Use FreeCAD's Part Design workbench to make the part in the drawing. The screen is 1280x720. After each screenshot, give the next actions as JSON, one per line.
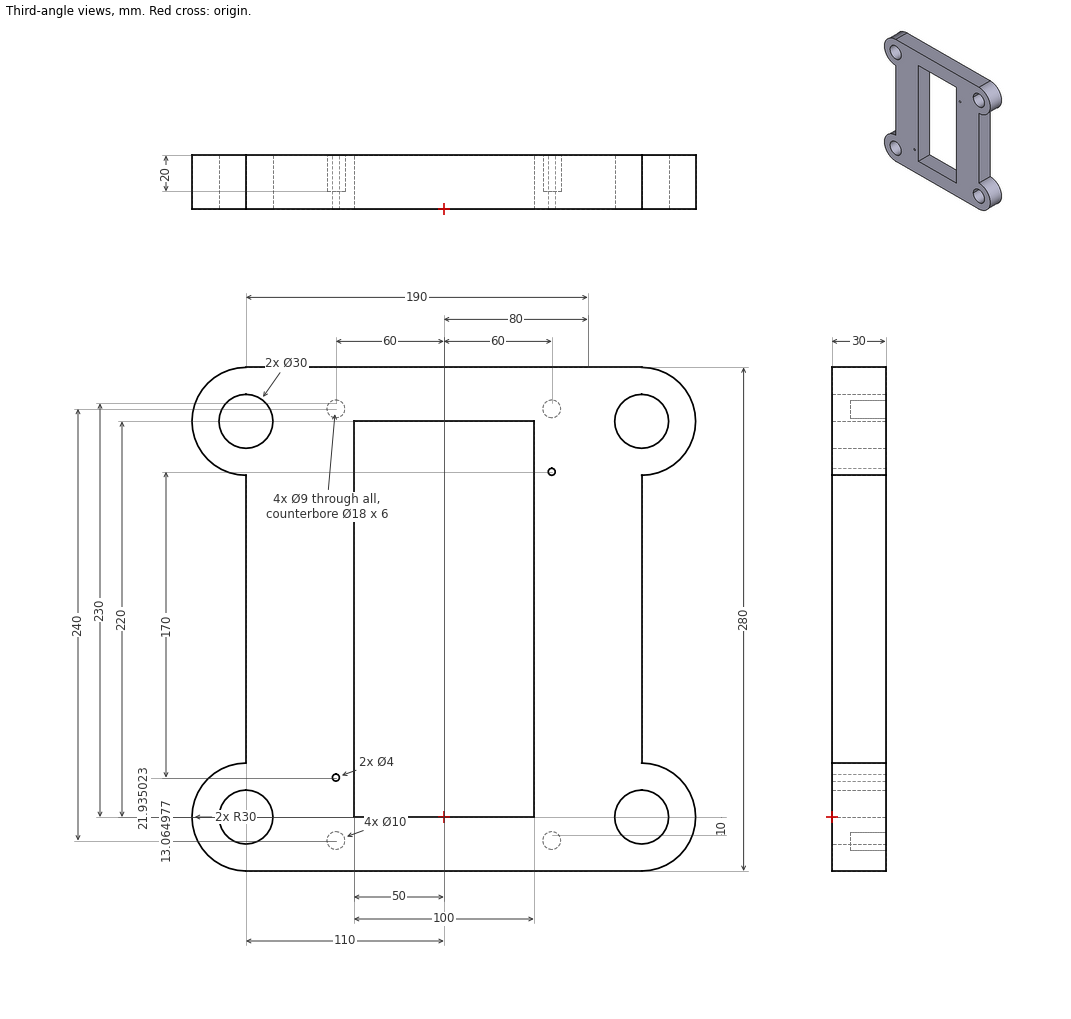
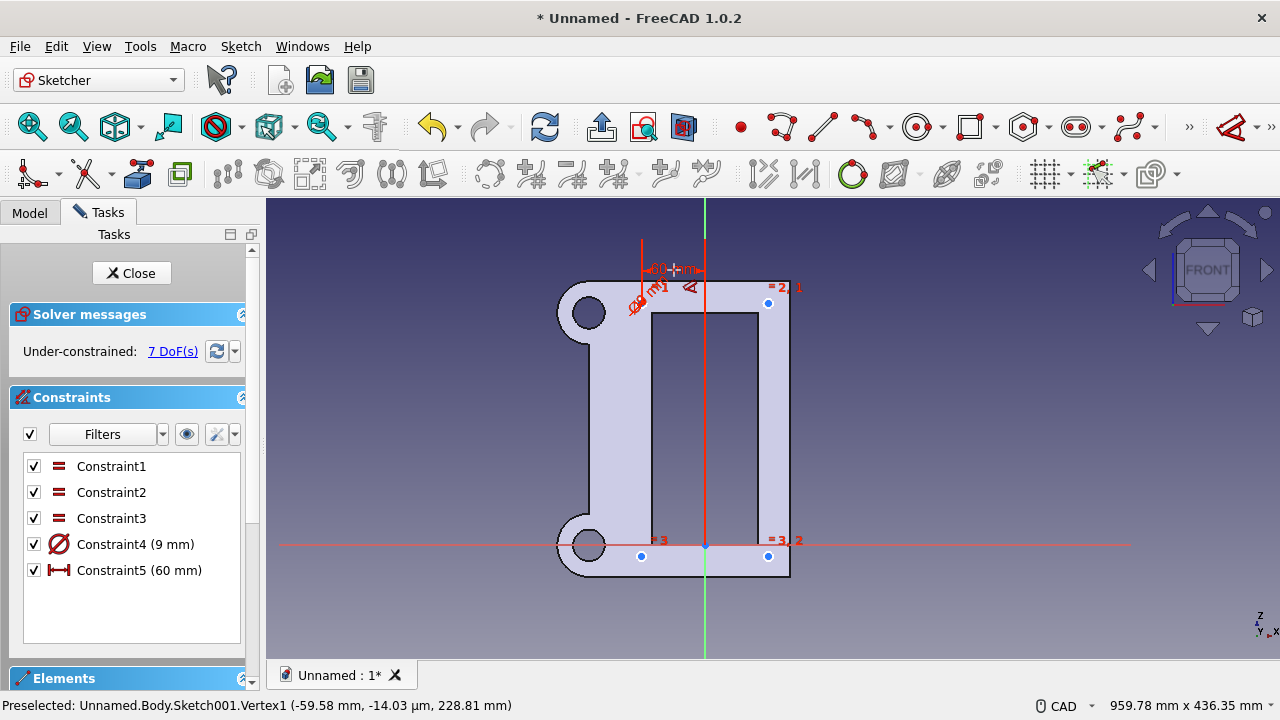
{"action": "left_click", "coordinate": [768, 304]}
{"action": "left_click", "coordinate": [751, 270]}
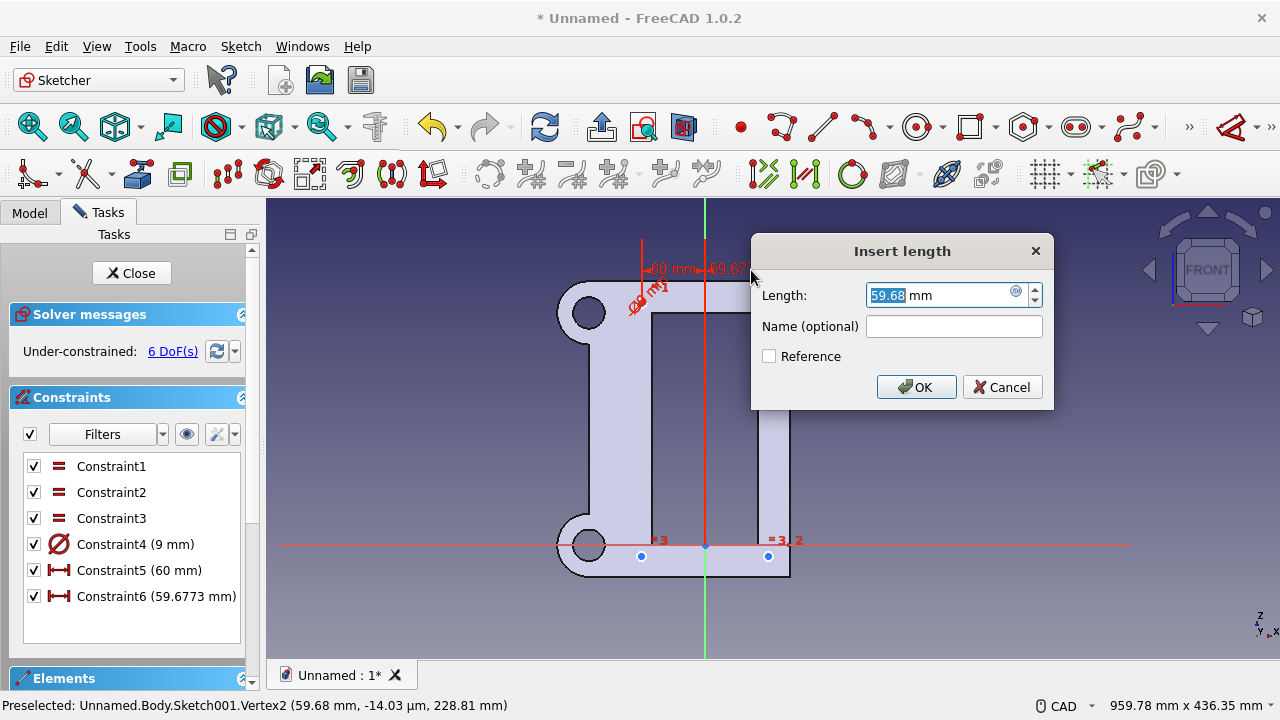
{"action": "type", "text": "60"}
{"action": "key", "text": "Return"}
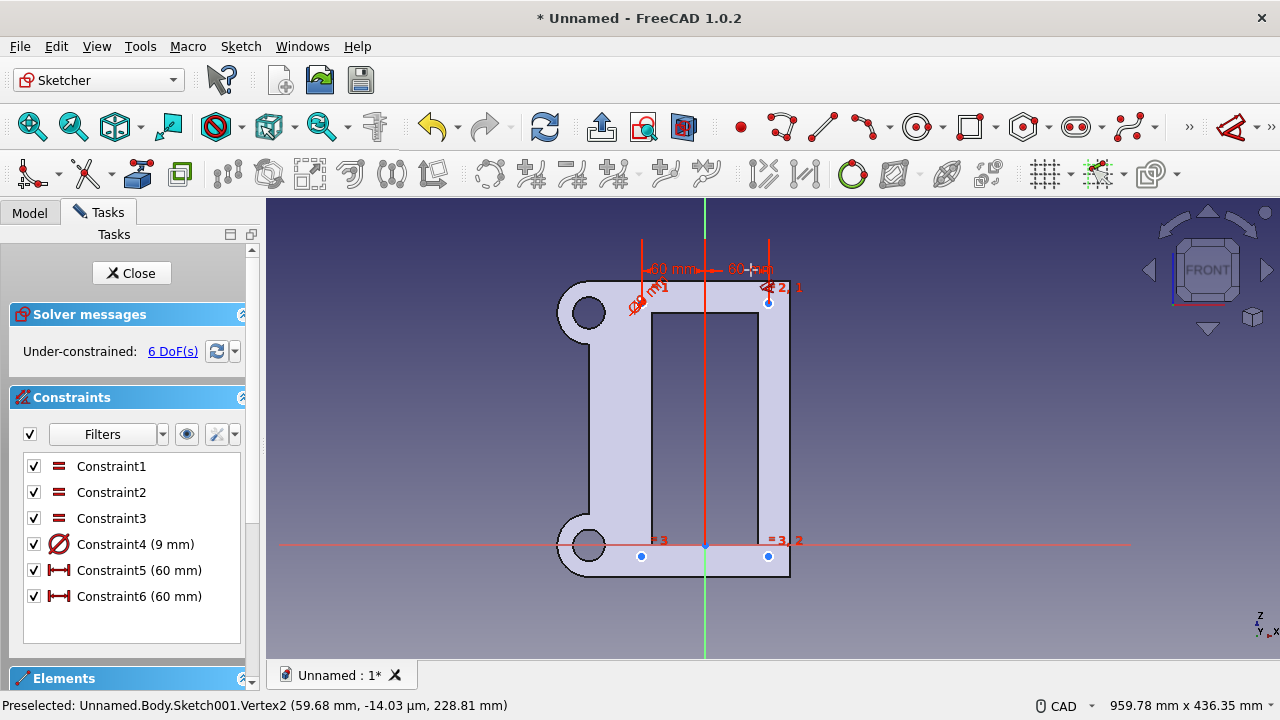
{"action": "left_click", "coordinate": [768, 557]}
{"action": "left_click", "coordinate": [737, 591]}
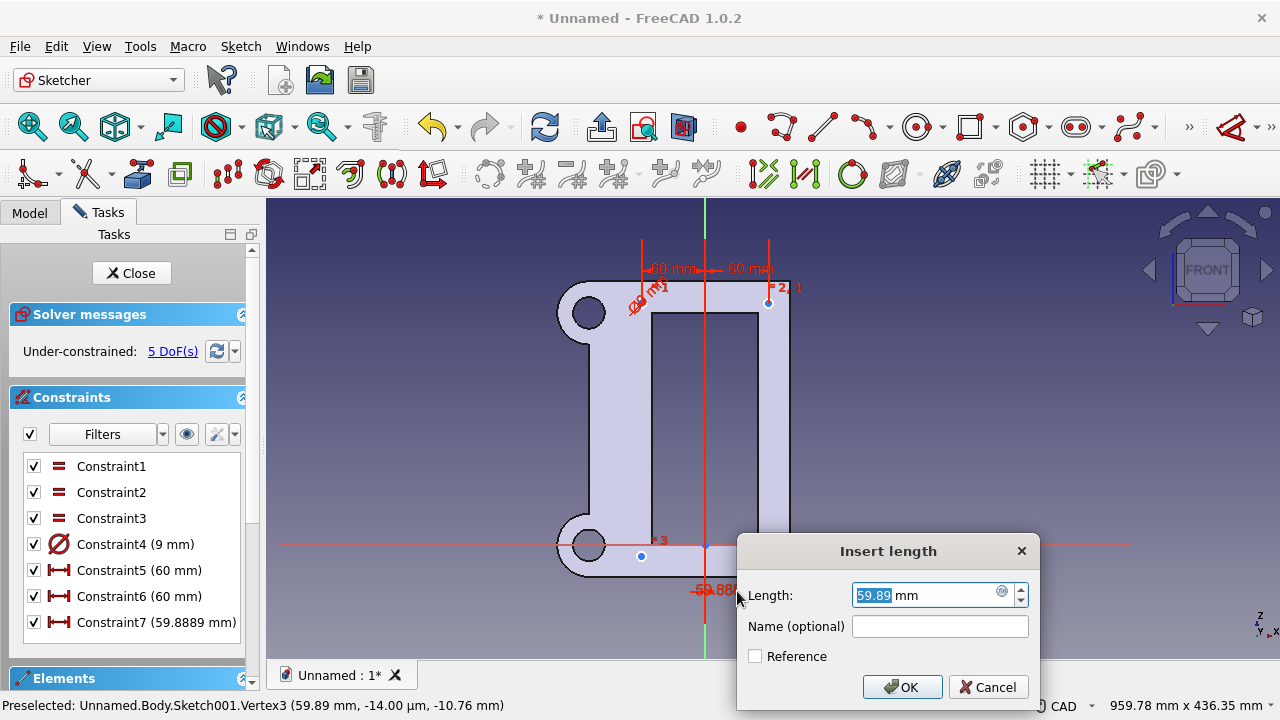
{"action": "type", "text": "60"}
{"action": "key", "text": "Return"}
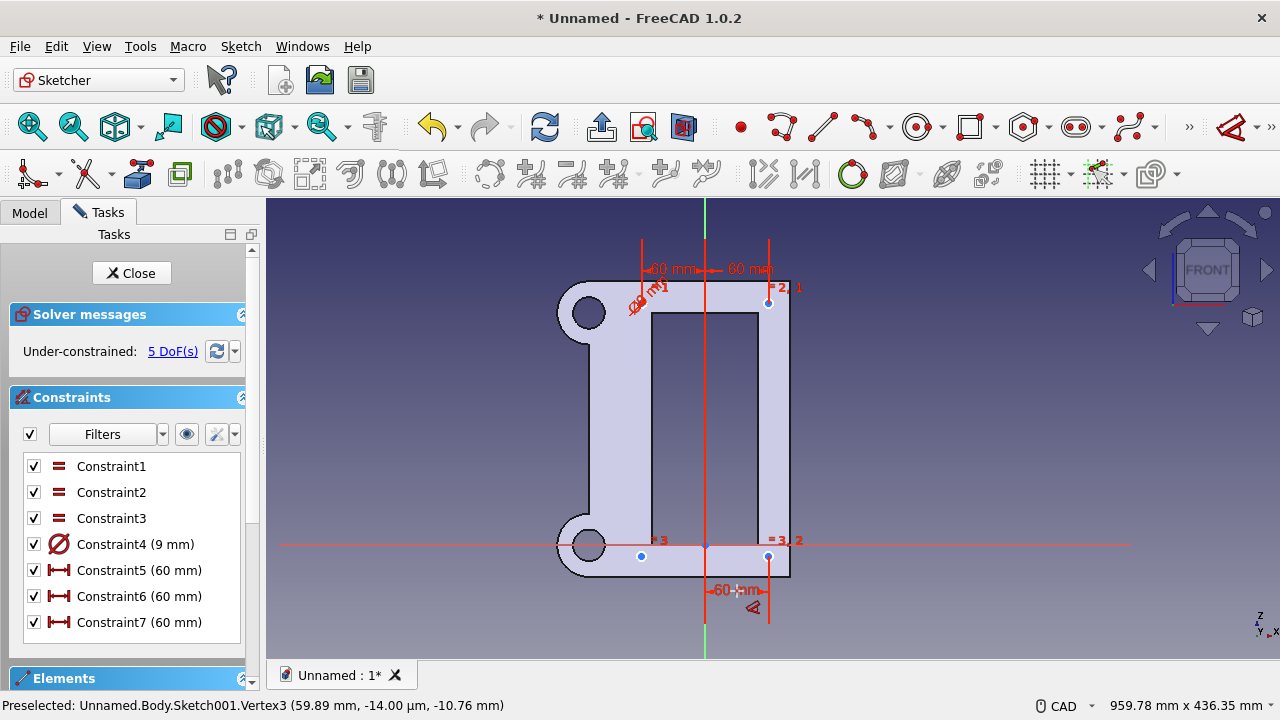
{"action": "scroll", "coordinate": [769, 557], "scroll_direction": "up", "scroll_amount": 7}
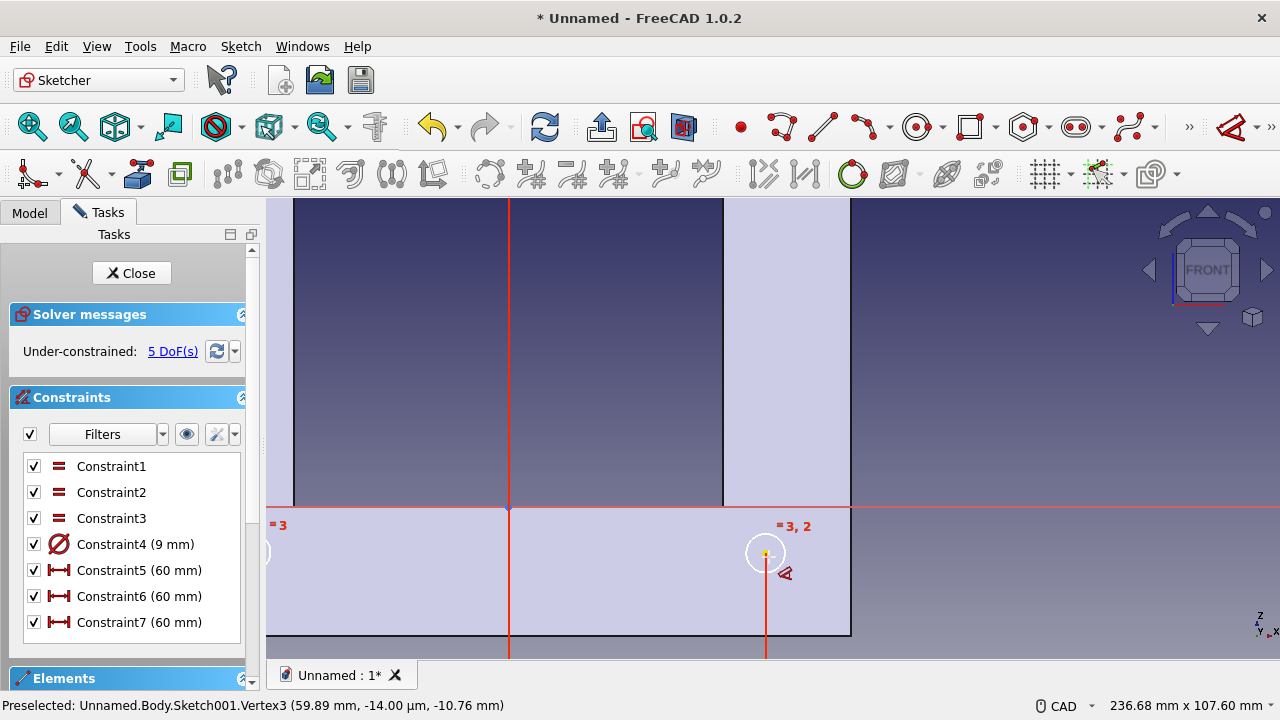
{"action": "left_click", "coordinate": [766, 553]}
{"action": "left_click", "coordinate": [800, 530]}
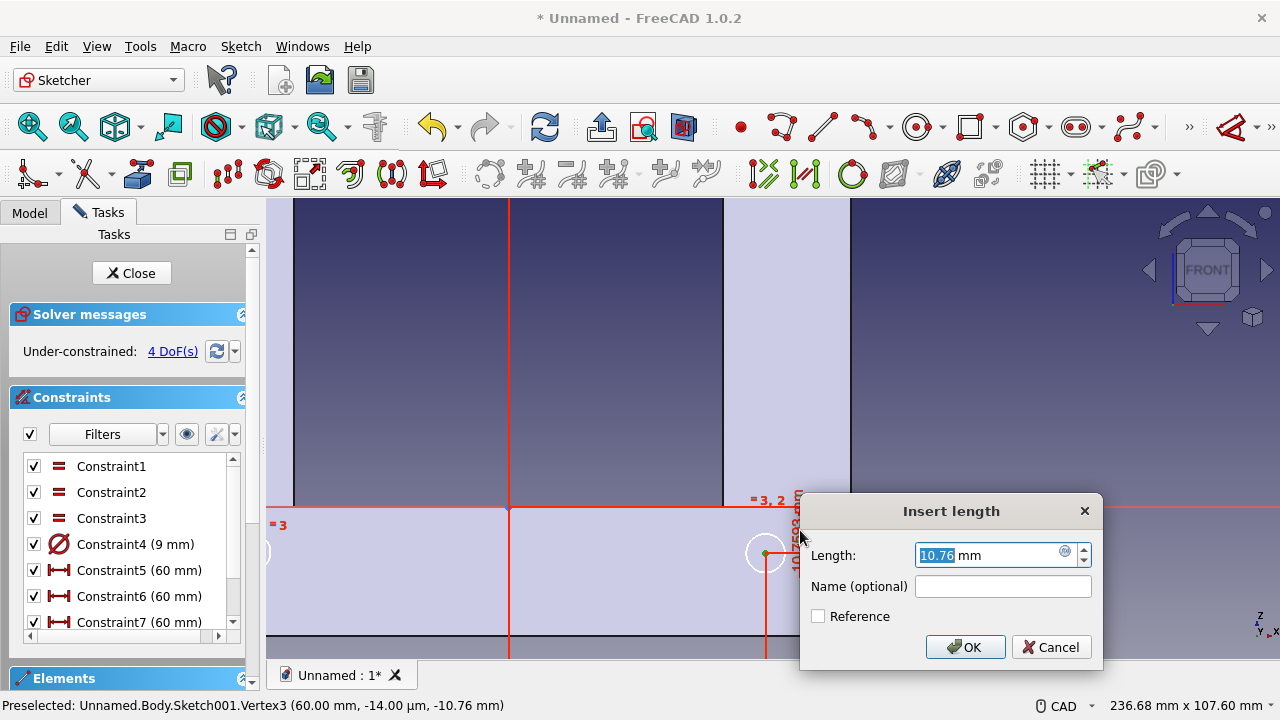
{"action": "type", "text": "10"}
{"action": "key", "text": "Return"}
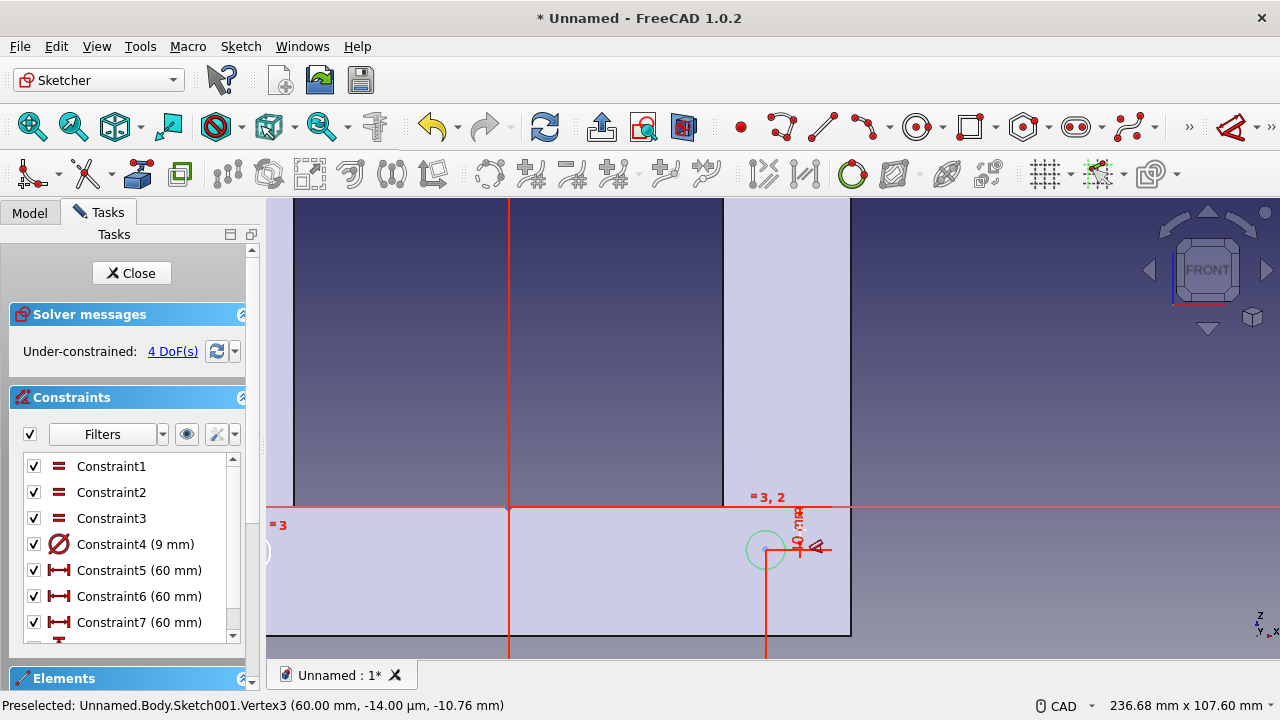
{"action": "scroll", "coordinate": [769, 557], "scroll_direction": "down", "scroll_amount": 7}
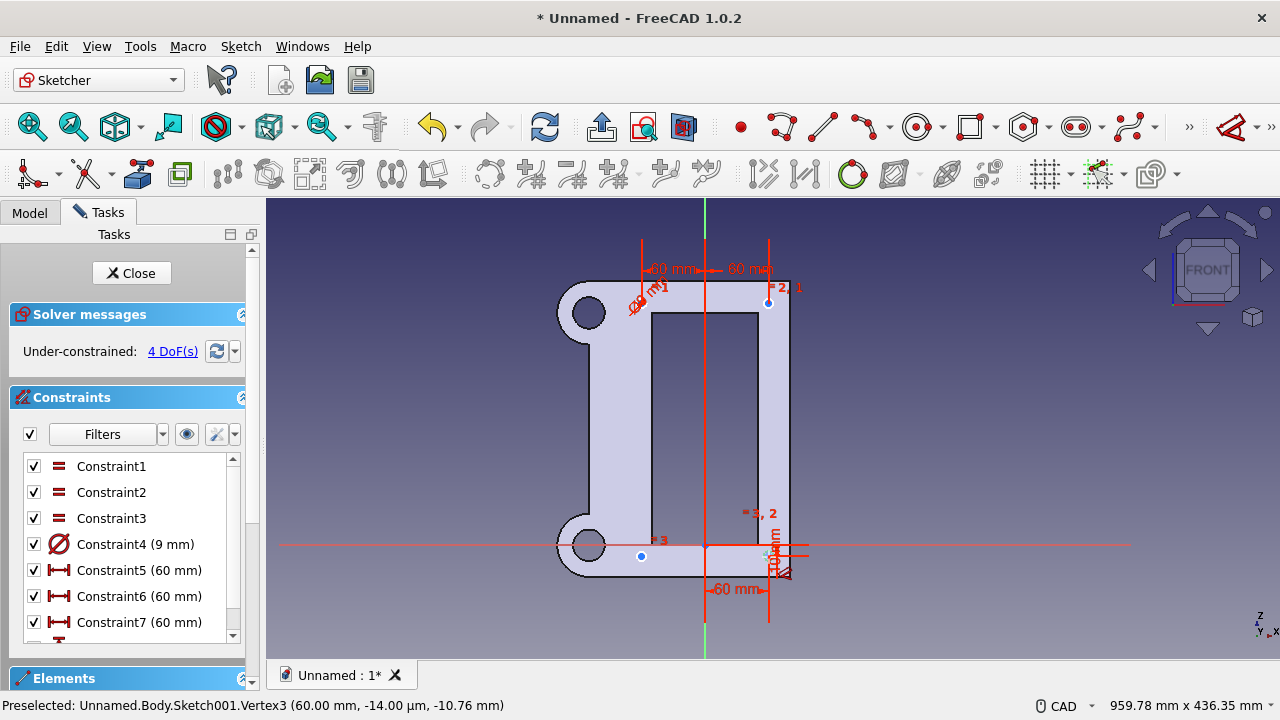
{"action": "left_click", "coordinate": [642, 556]}
{"action": "left_click", "coordinate": [659, 590]}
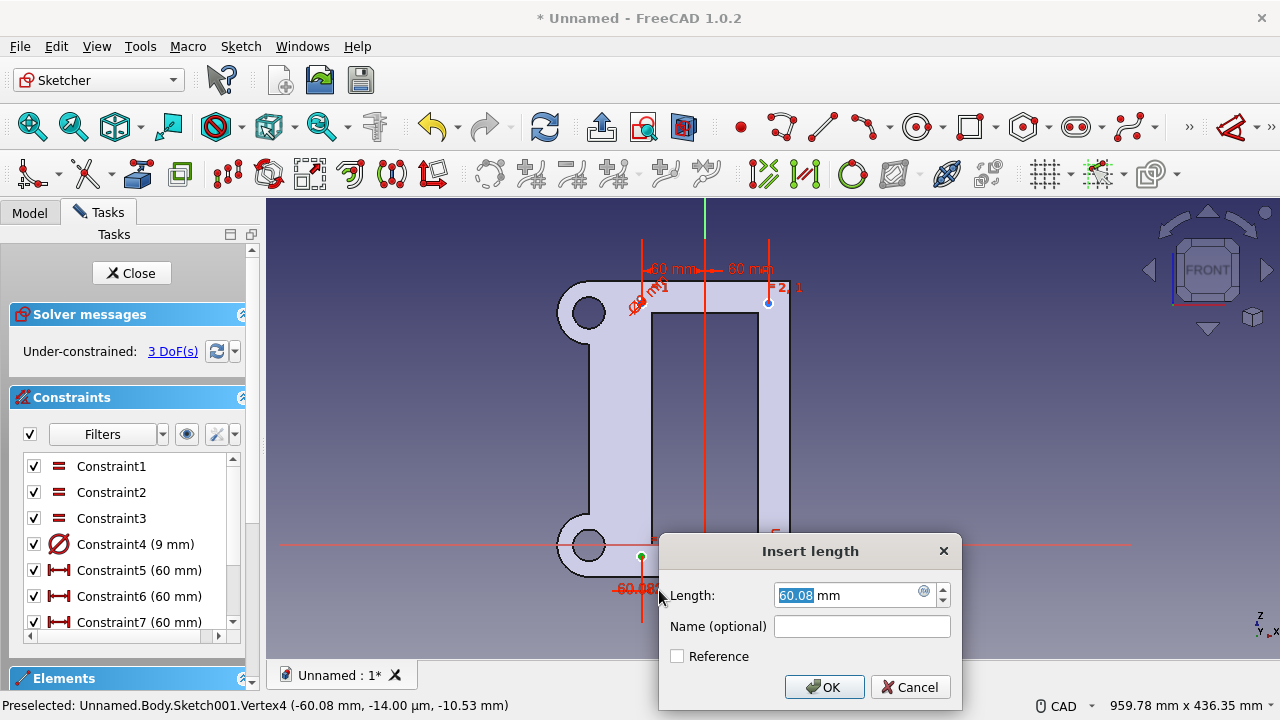
{"action": "type", "text": "60"}
{"action": "key", "text": "Return"}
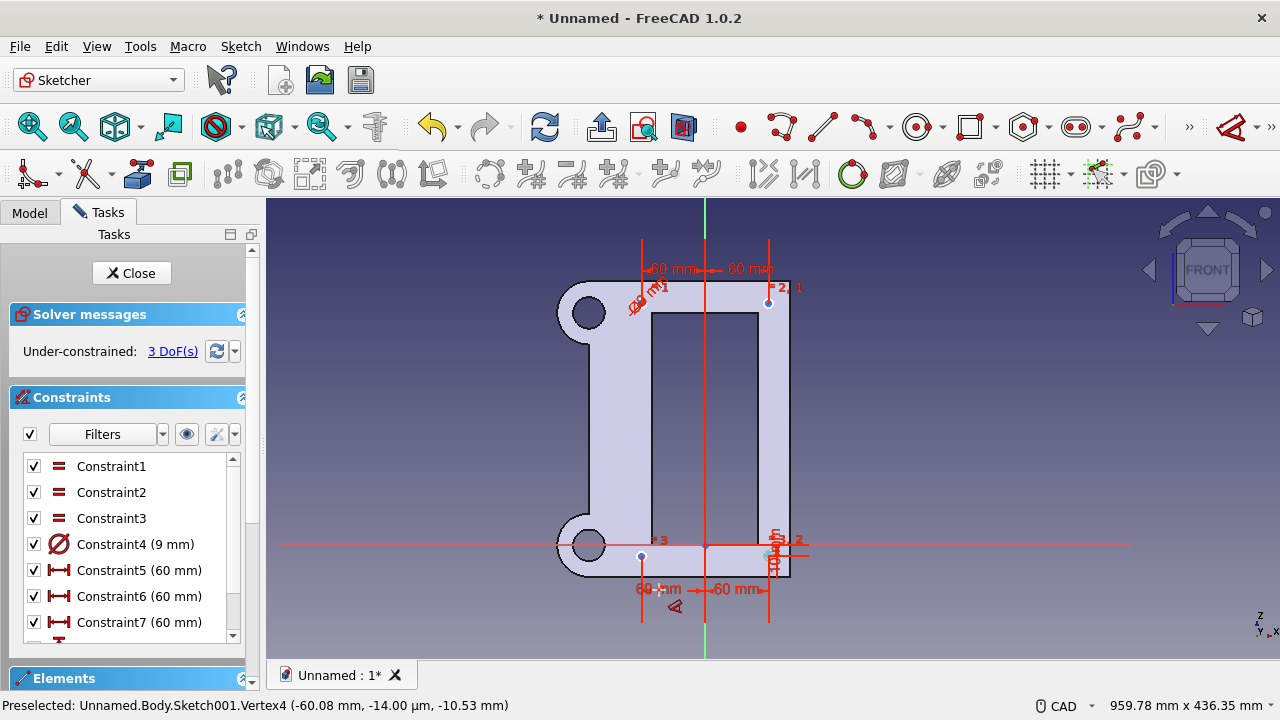
{"action": "scroll", "coordinate": [642, 556], "scroll_direction": "up", "scroll_amount": 7}